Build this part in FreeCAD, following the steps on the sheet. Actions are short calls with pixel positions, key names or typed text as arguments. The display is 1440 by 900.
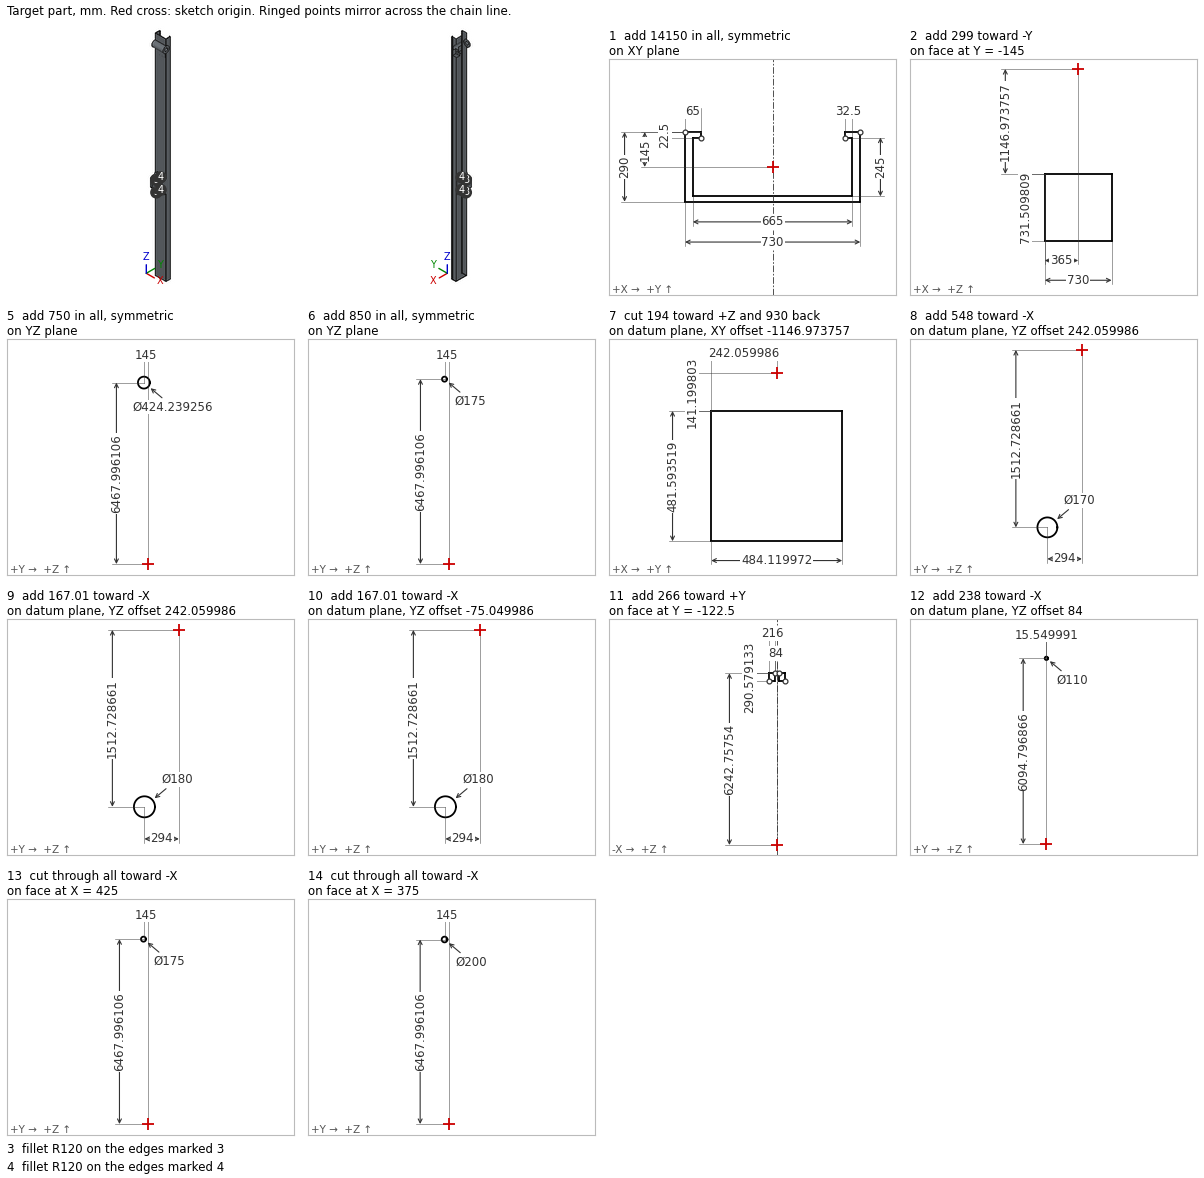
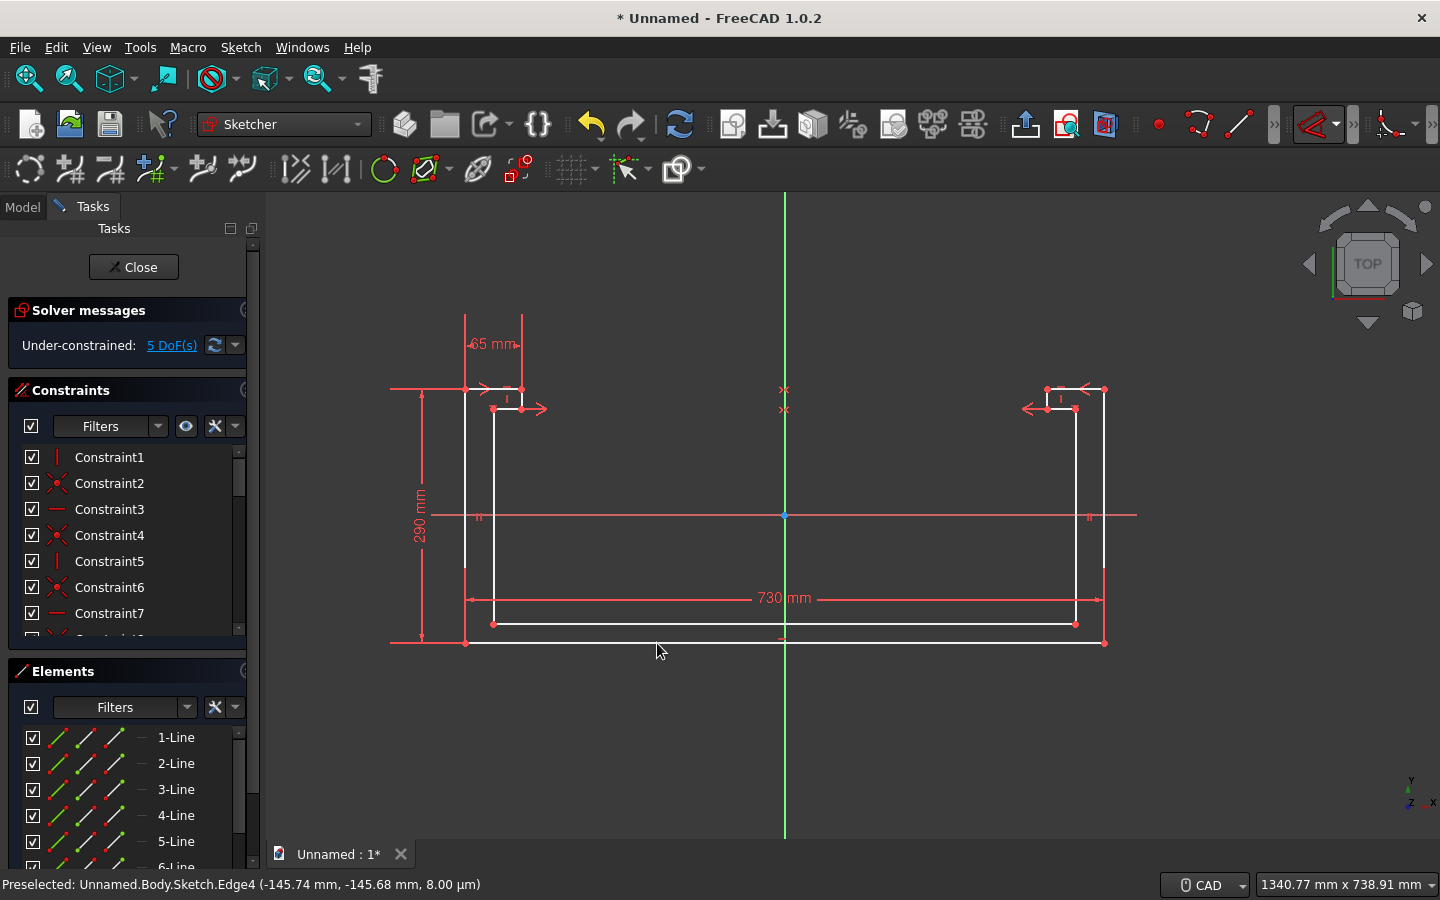
click(1076, 474)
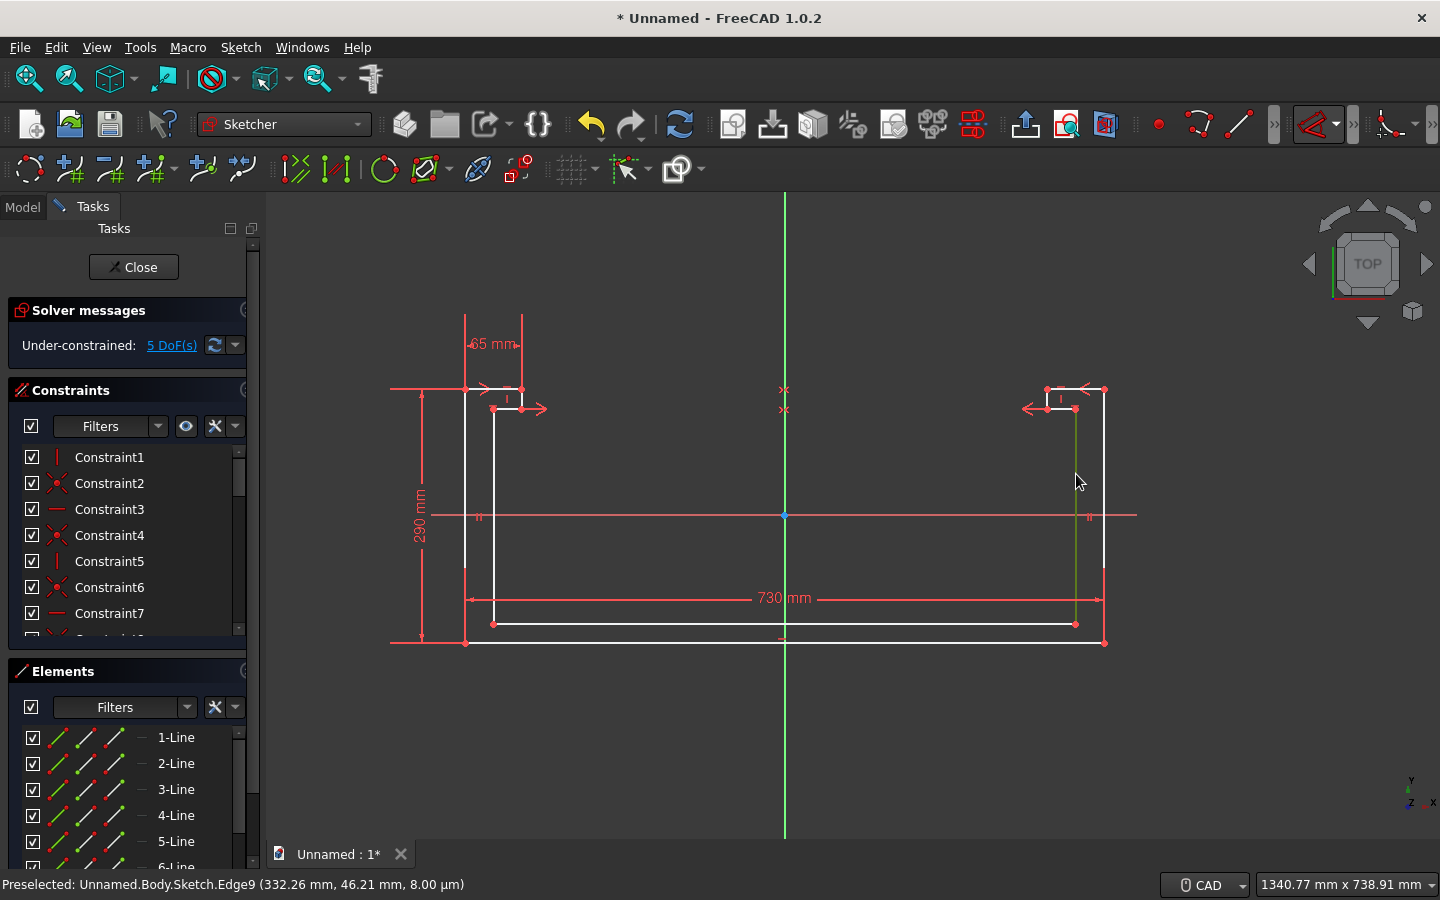
key(i)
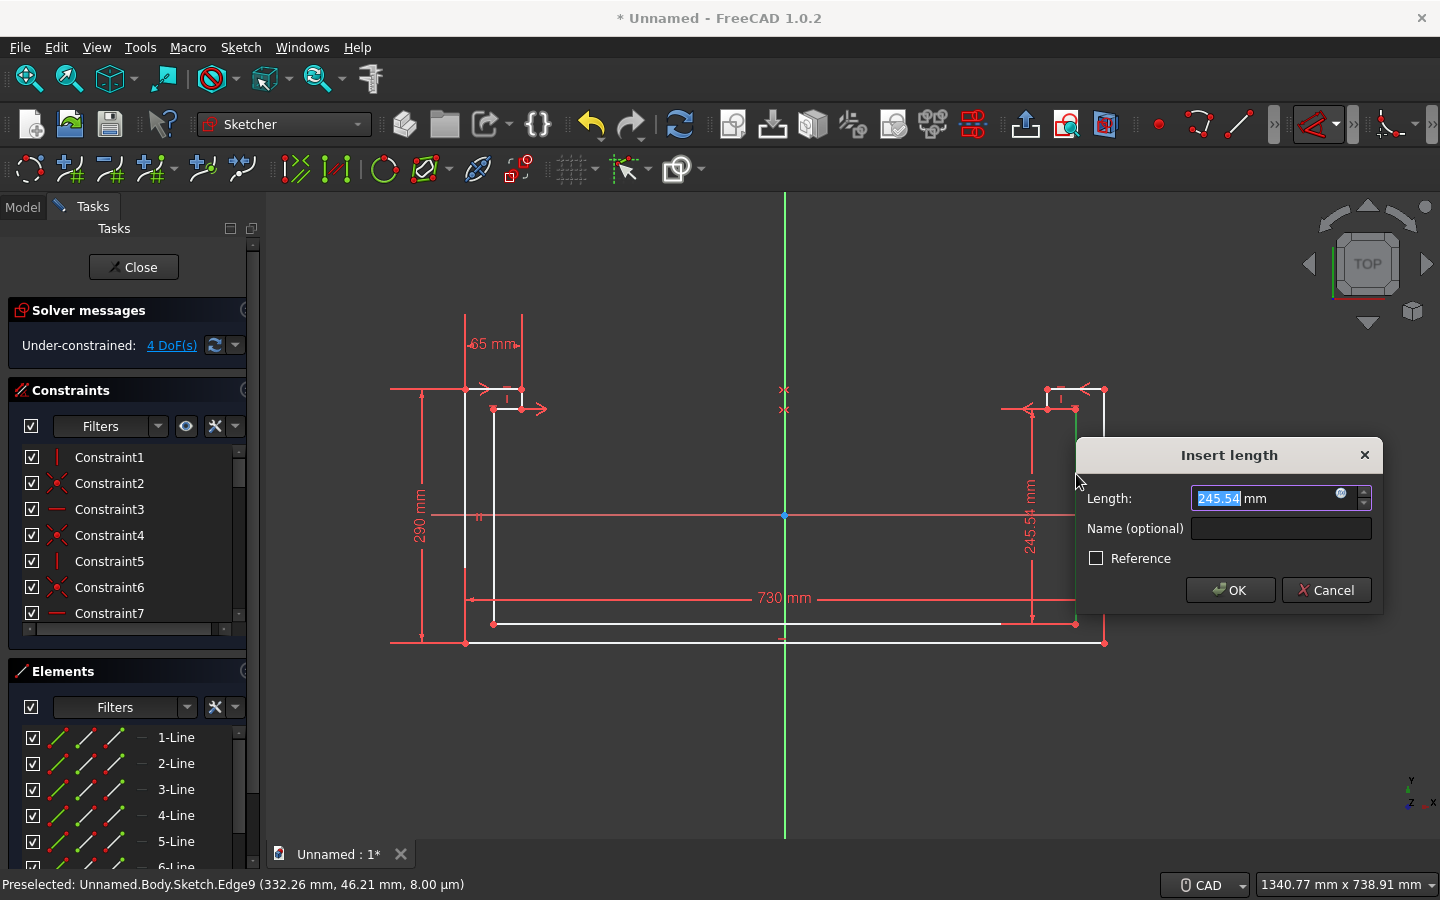
text(245)
key(Return)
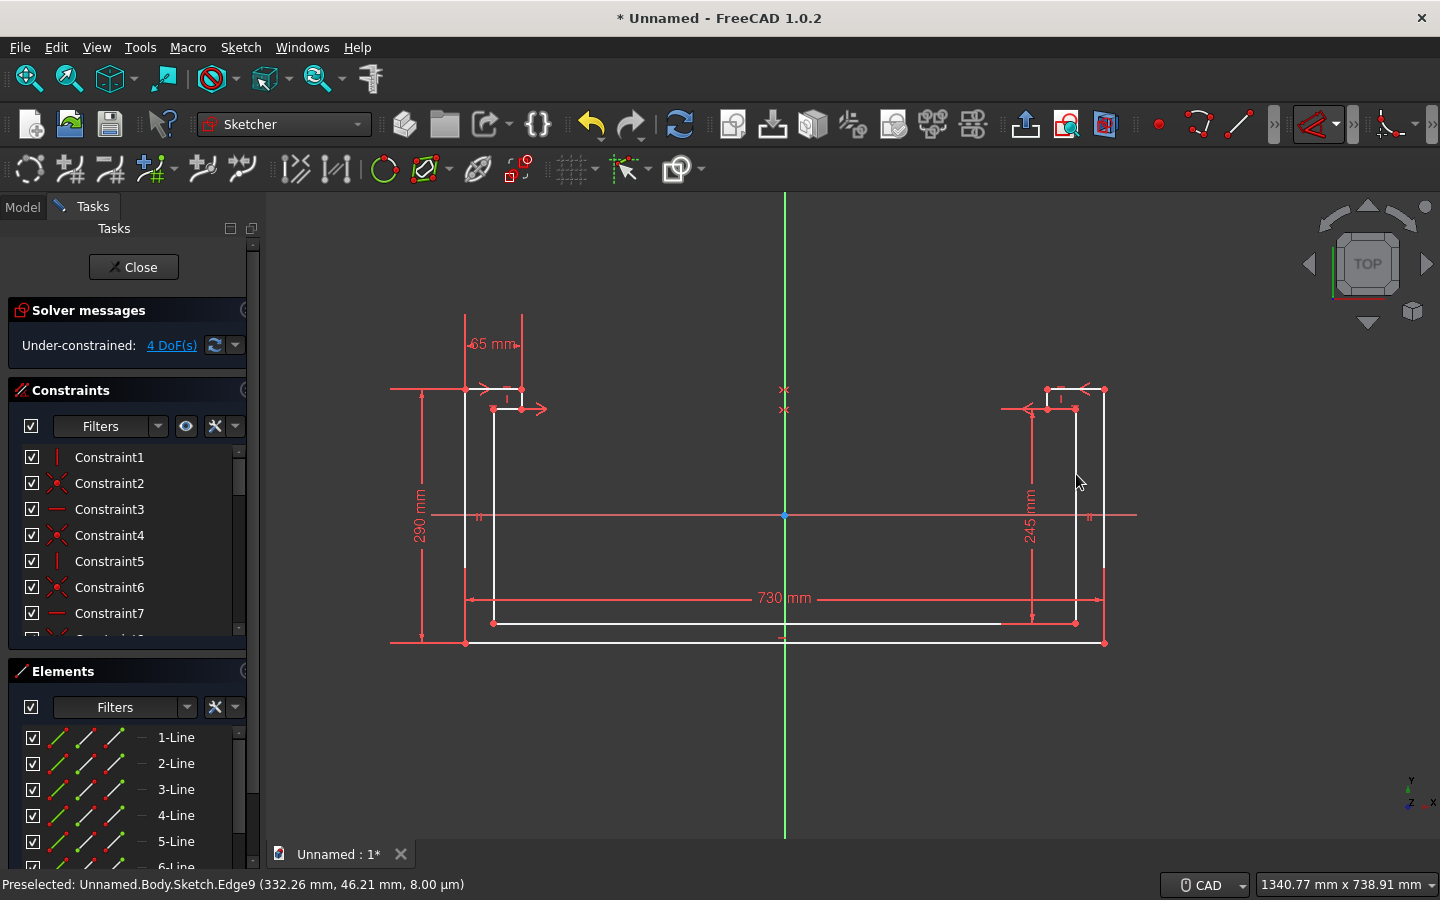
click(901, 624)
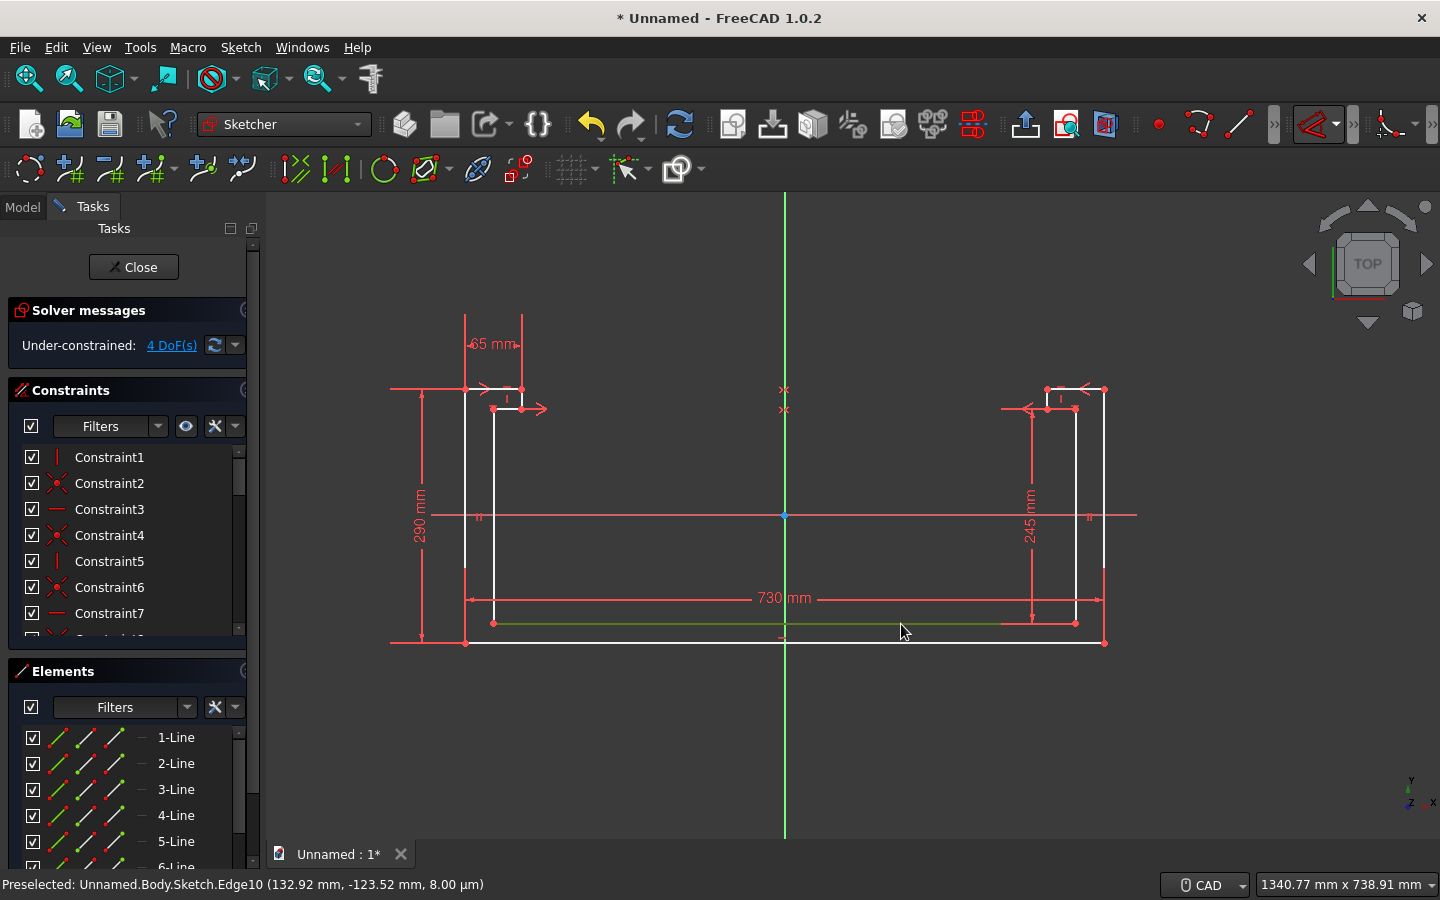
key(l)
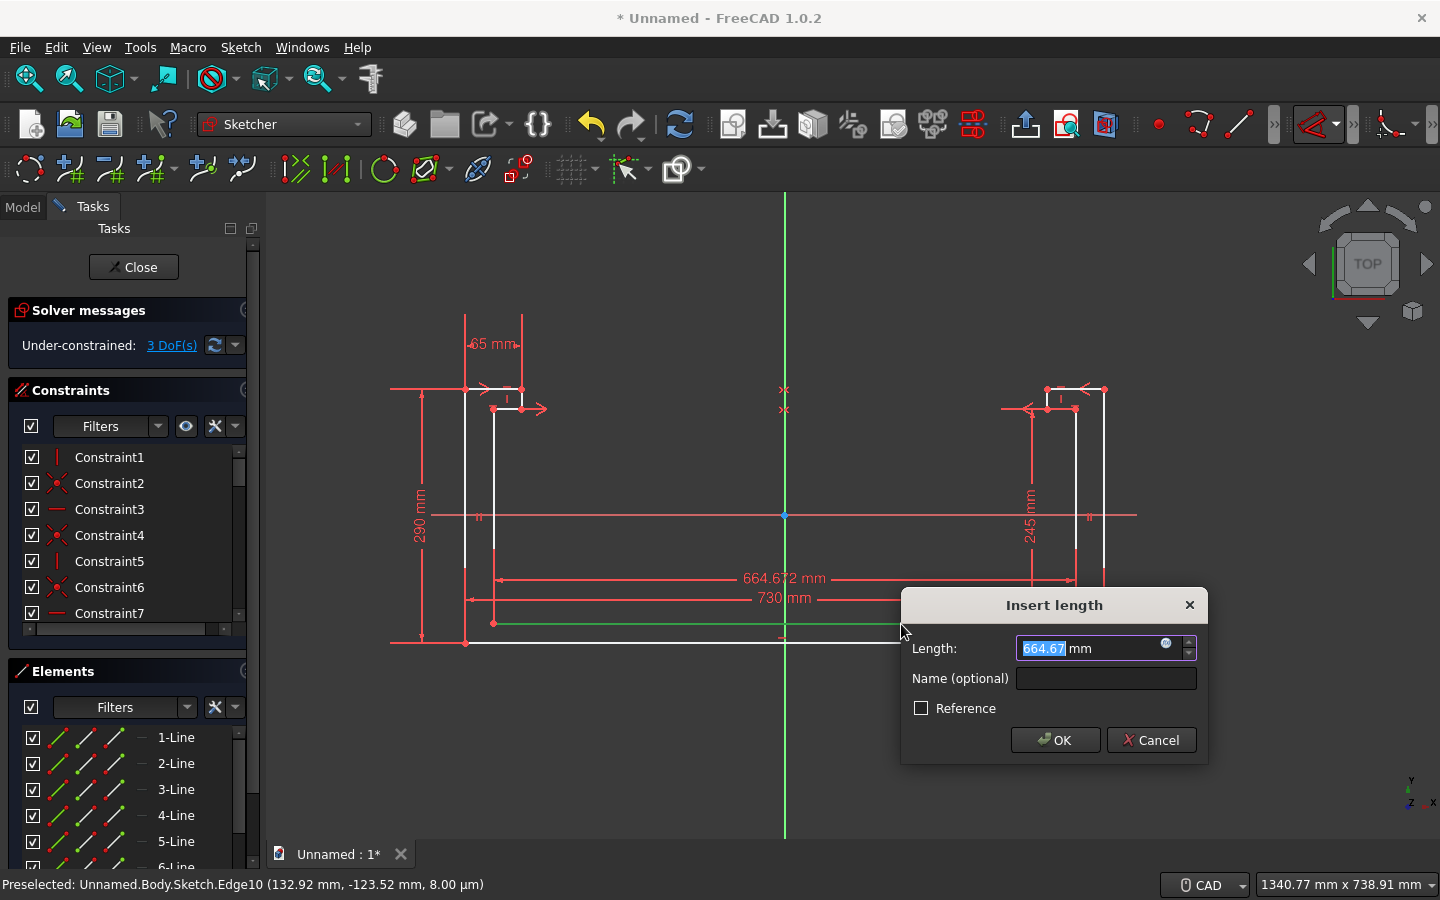
text(665)
key(Return)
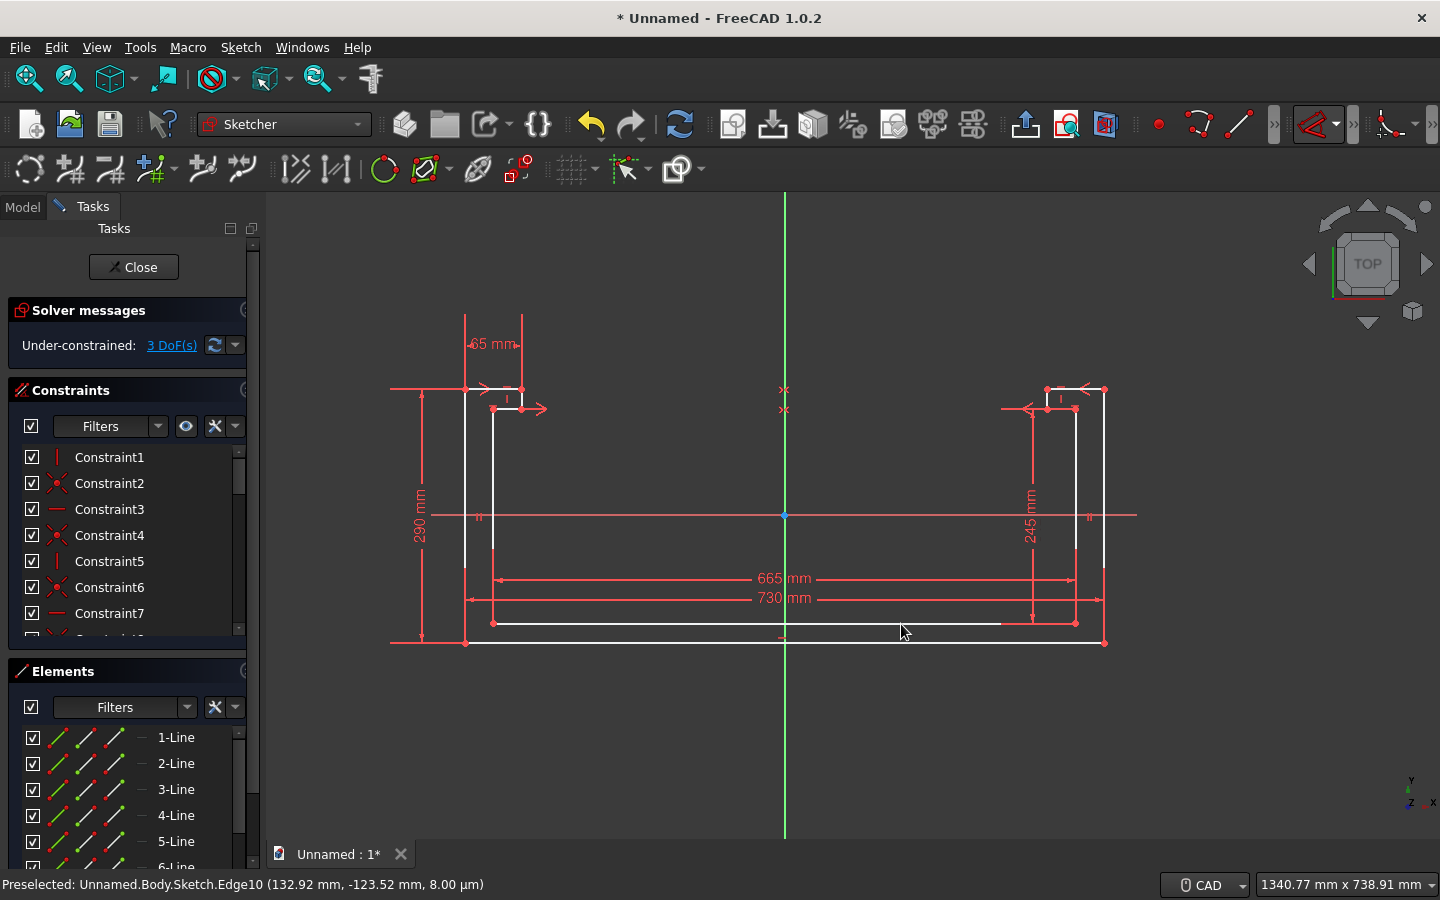
scroll(522, 399, up, 4)